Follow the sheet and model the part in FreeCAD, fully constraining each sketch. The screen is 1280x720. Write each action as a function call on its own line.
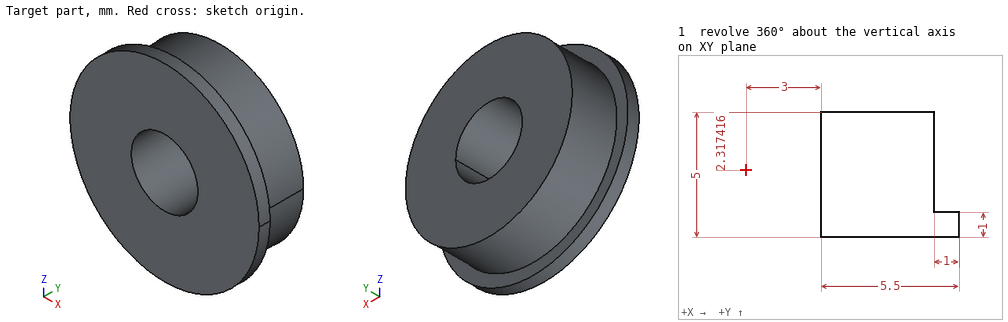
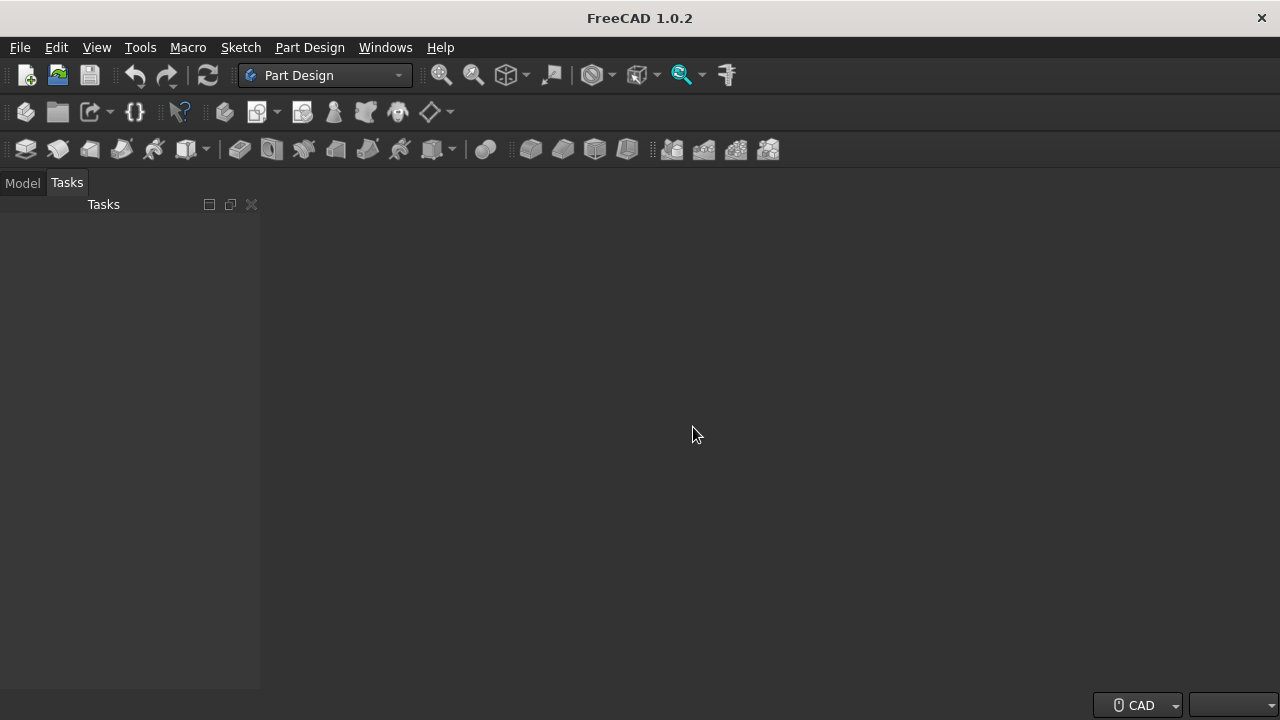
click(26, 76)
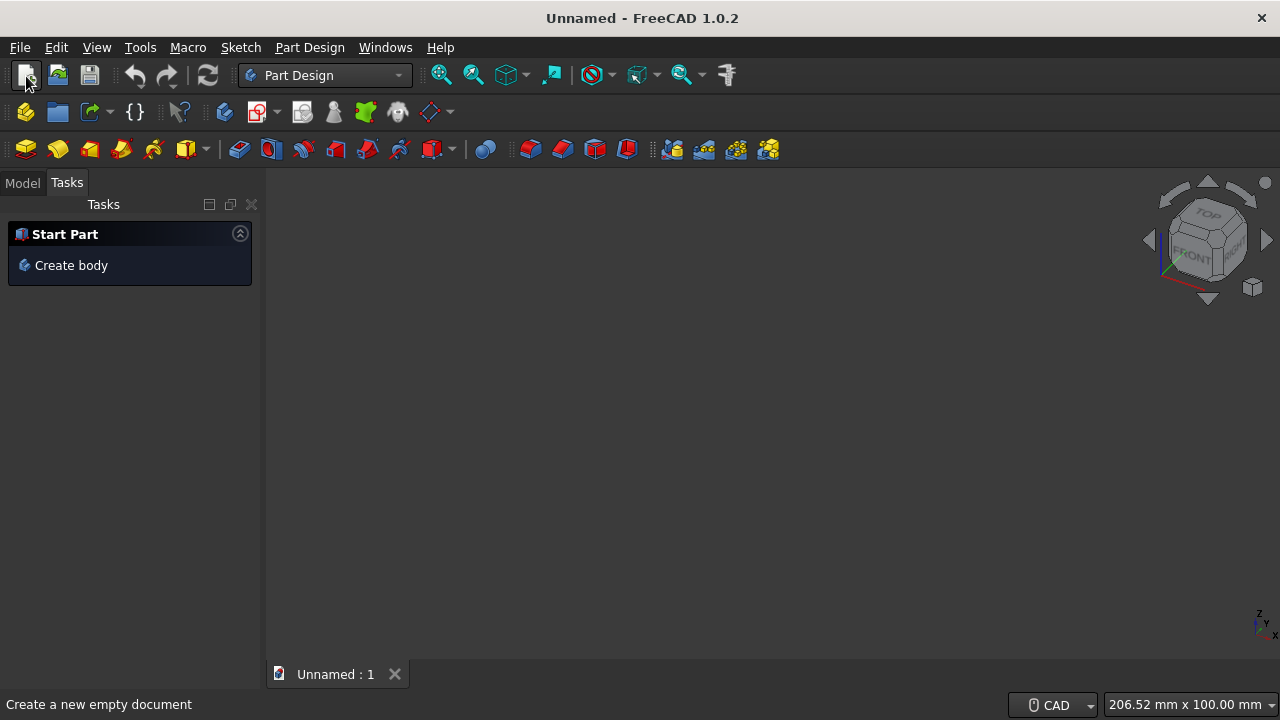
click(258, 112)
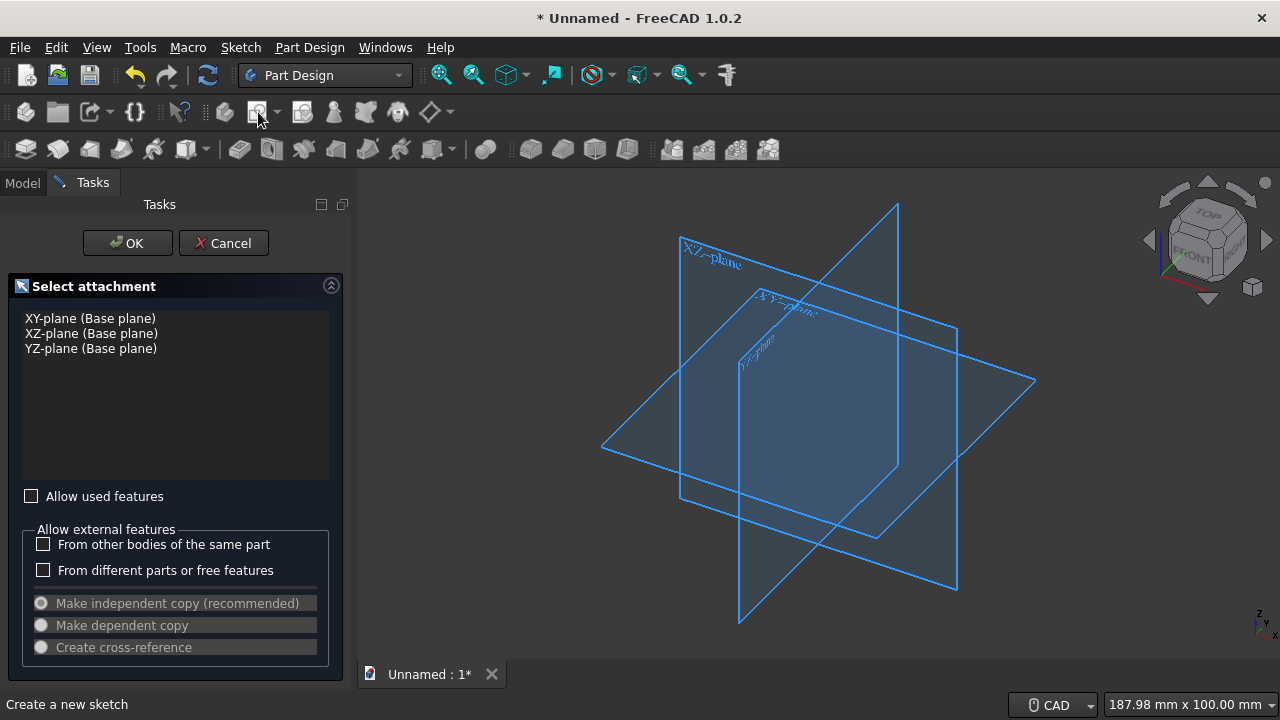
click(82, 318)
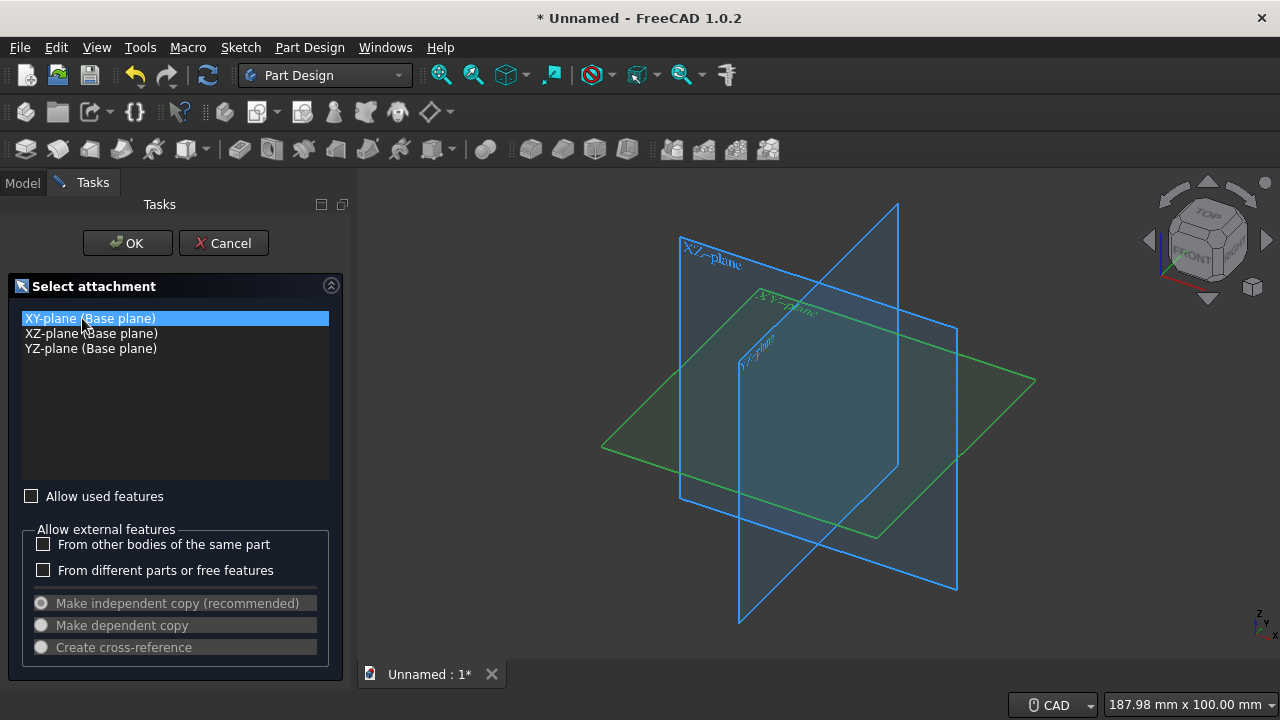
click(128, 243)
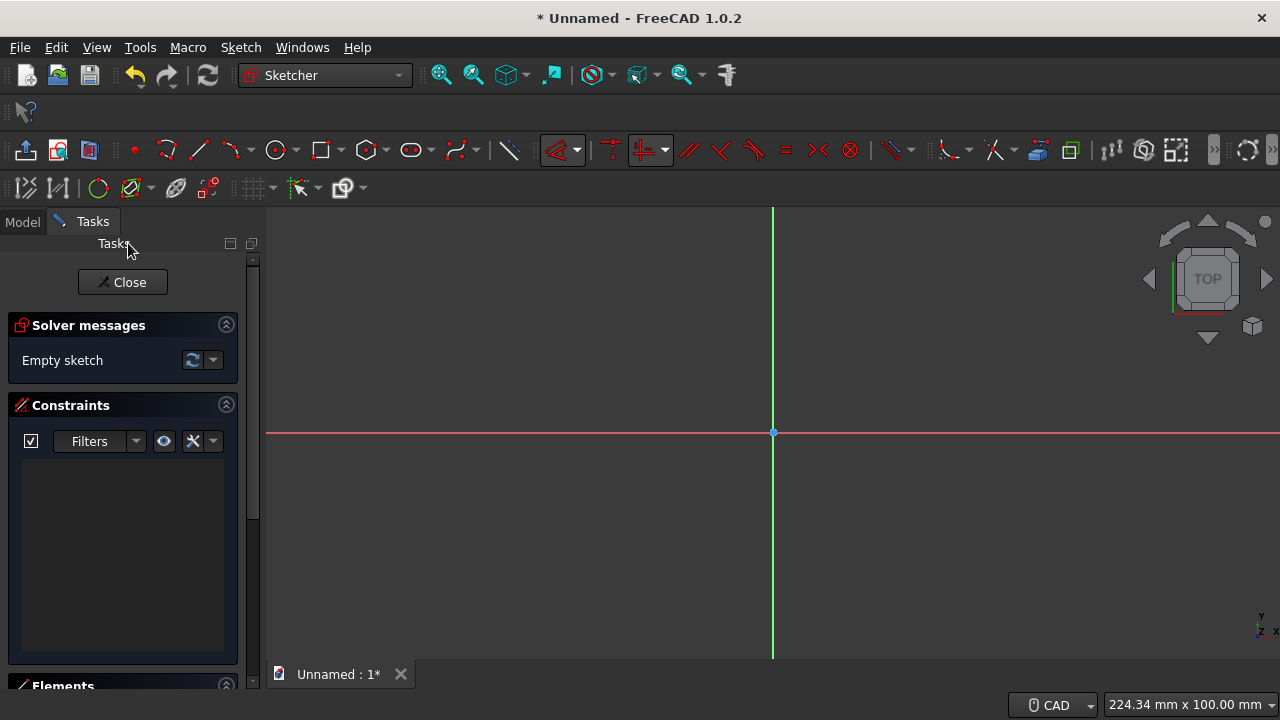
scroll(799, 434, up, 13)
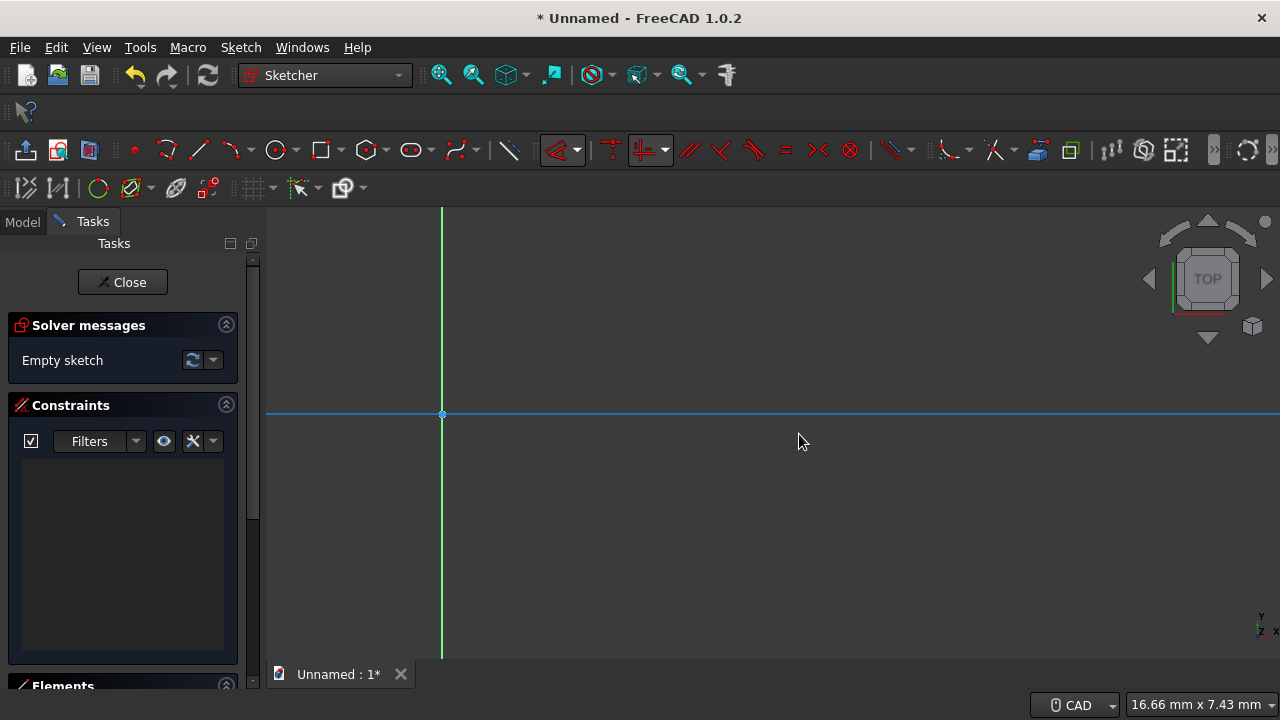
click(168, 150)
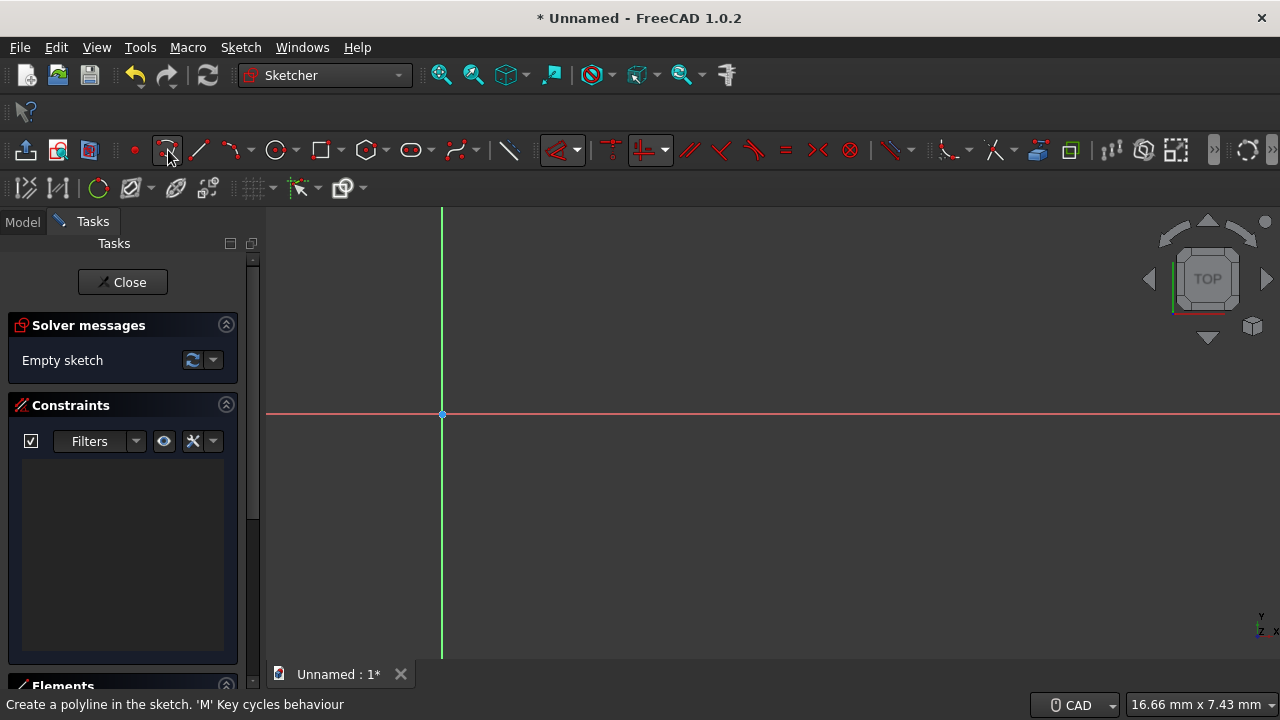
click(625, 273)
click(625, 578)
click(960, 578)
click(960, 517)
click(899, 517)
click(899, 273)
click(625, 274)
key(Escape)
key(Escape)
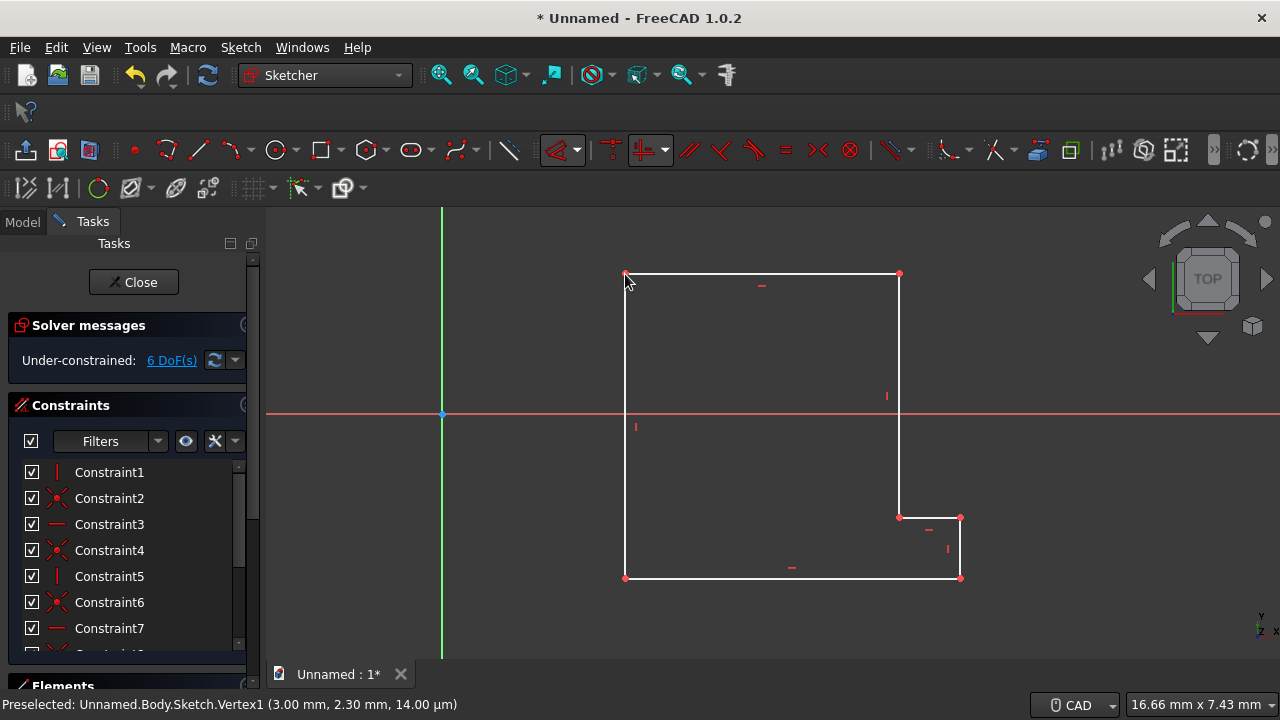
click(556, 150)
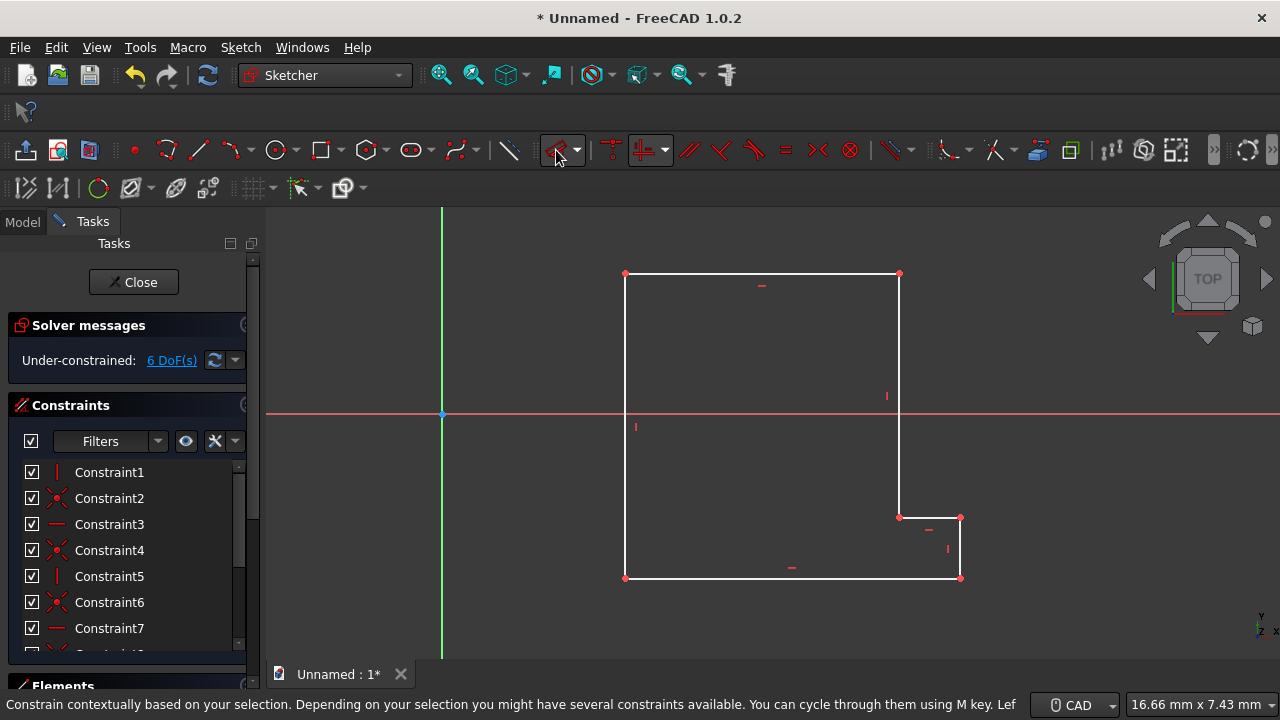
click(625, 365)
click(591, 356)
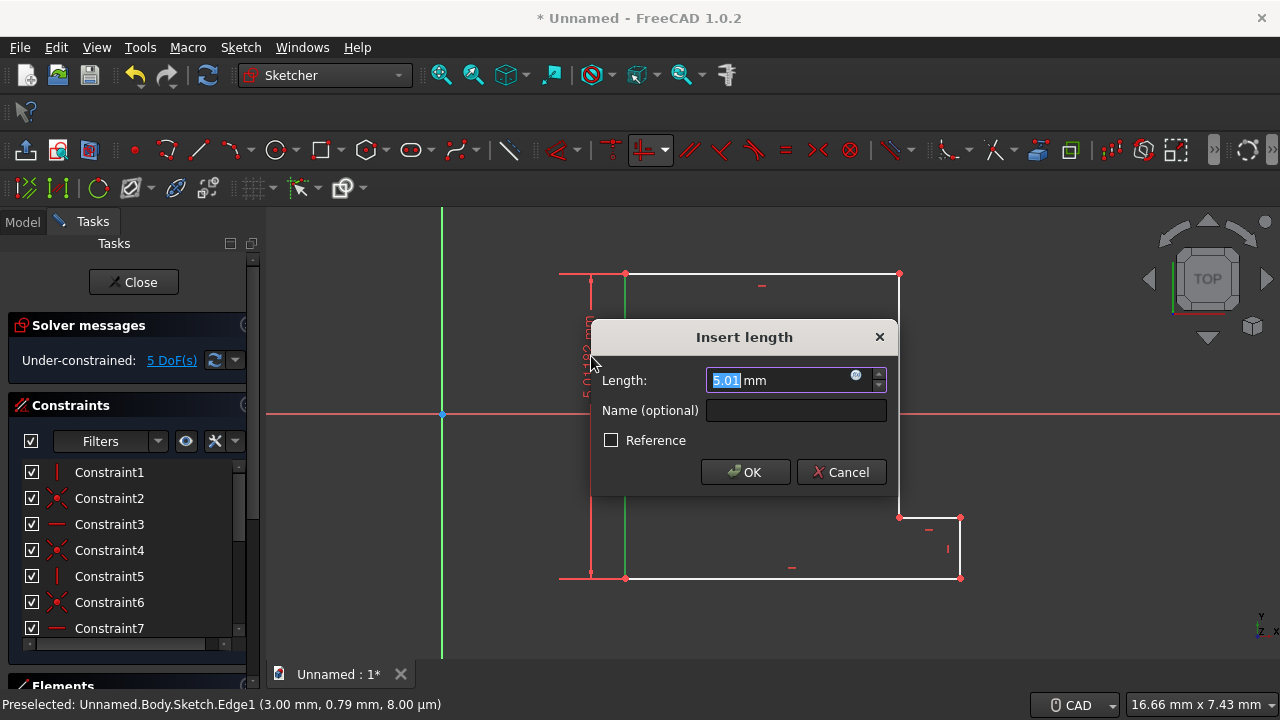
text(5)
key(Return)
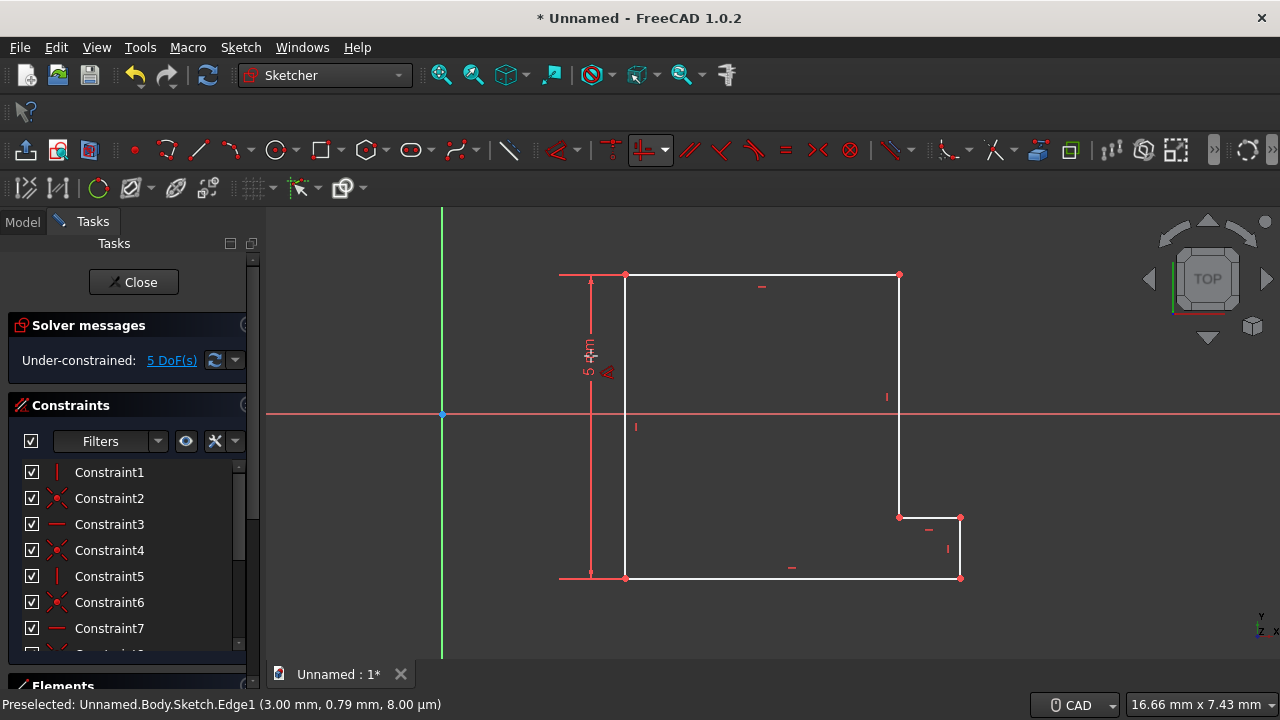
click(960, 561)
click(994, 549)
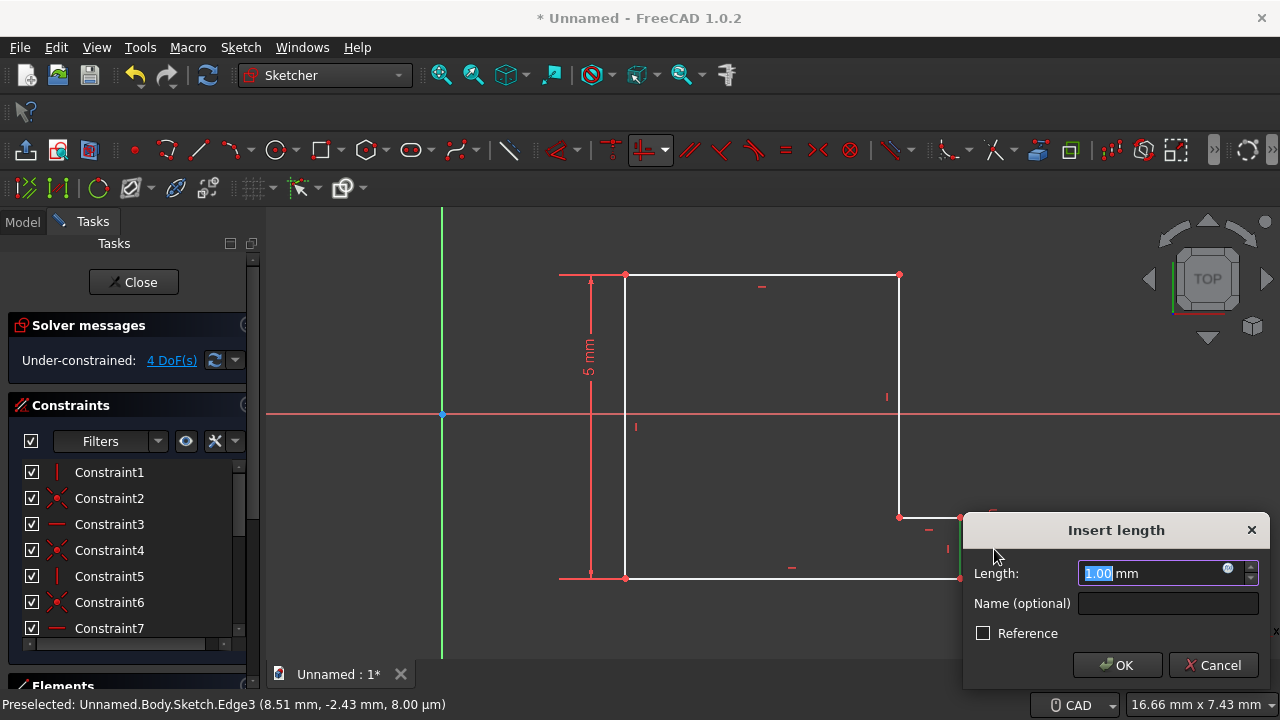
text(1)
key(Return)